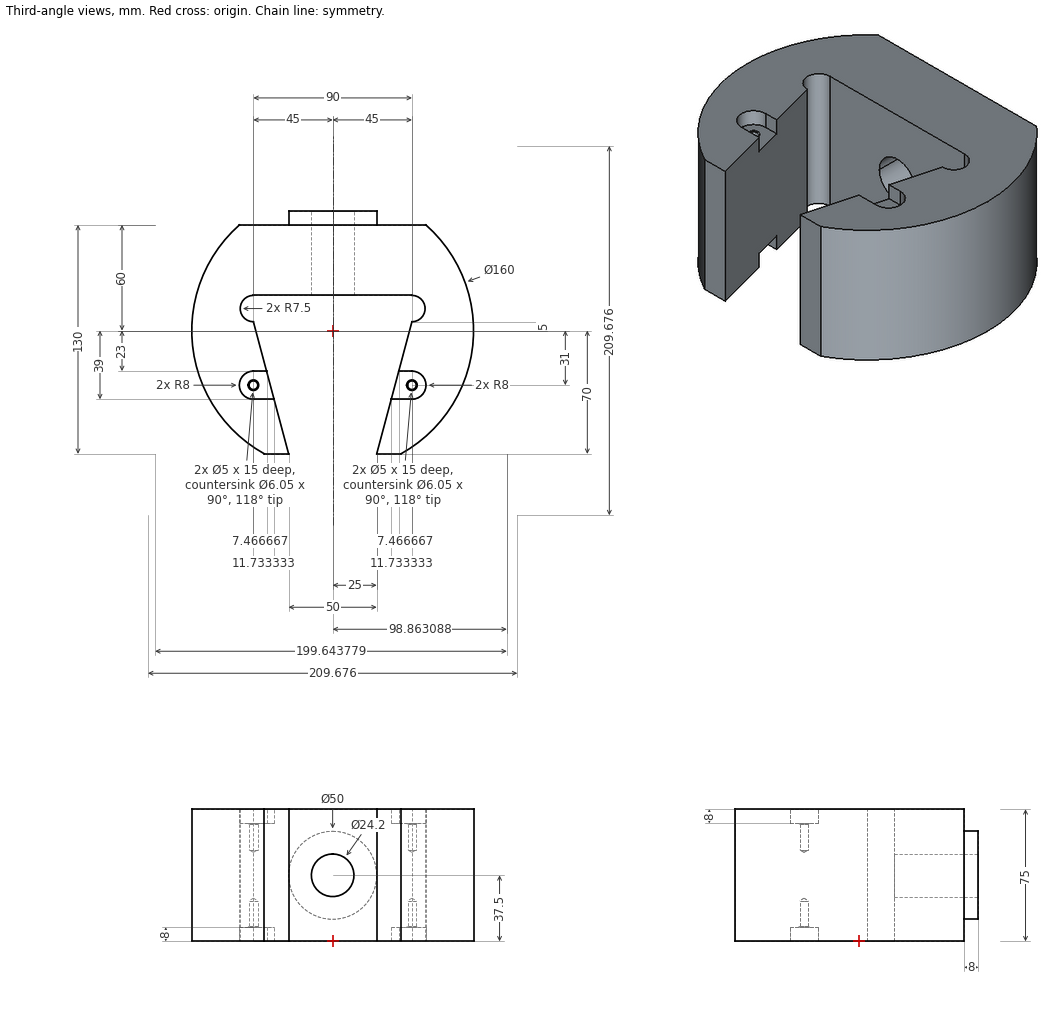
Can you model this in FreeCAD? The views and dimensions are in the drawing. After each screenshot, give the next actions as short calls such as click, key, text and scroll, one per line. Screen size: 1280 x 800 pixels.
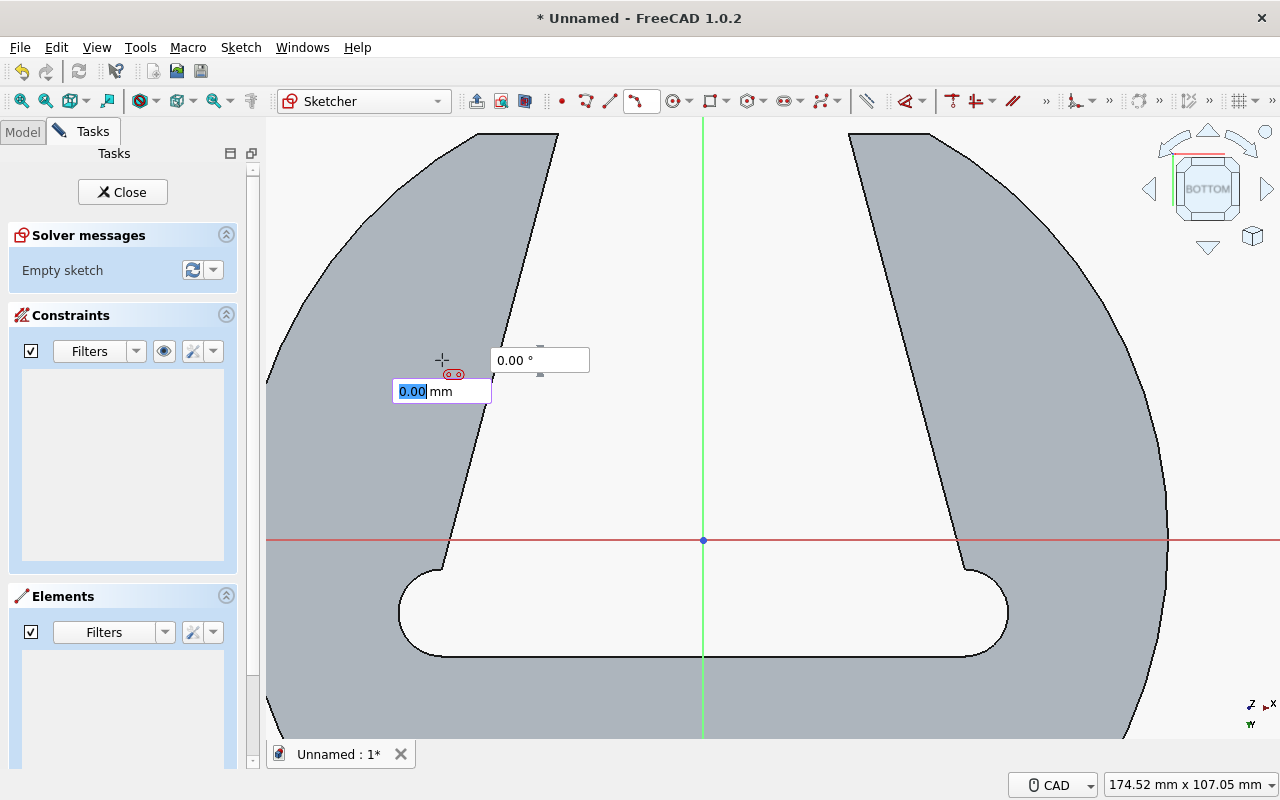
click(965, 360)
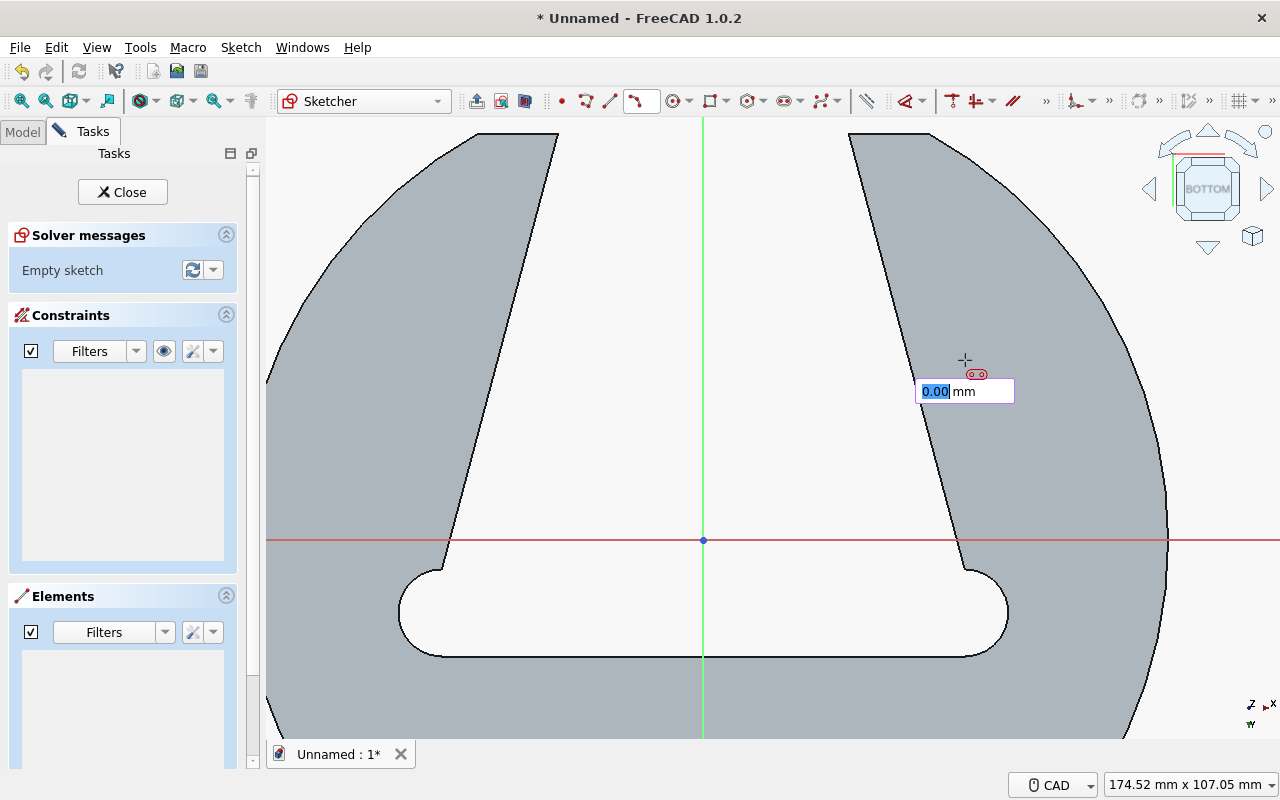
click(625, 407)
key(Escape)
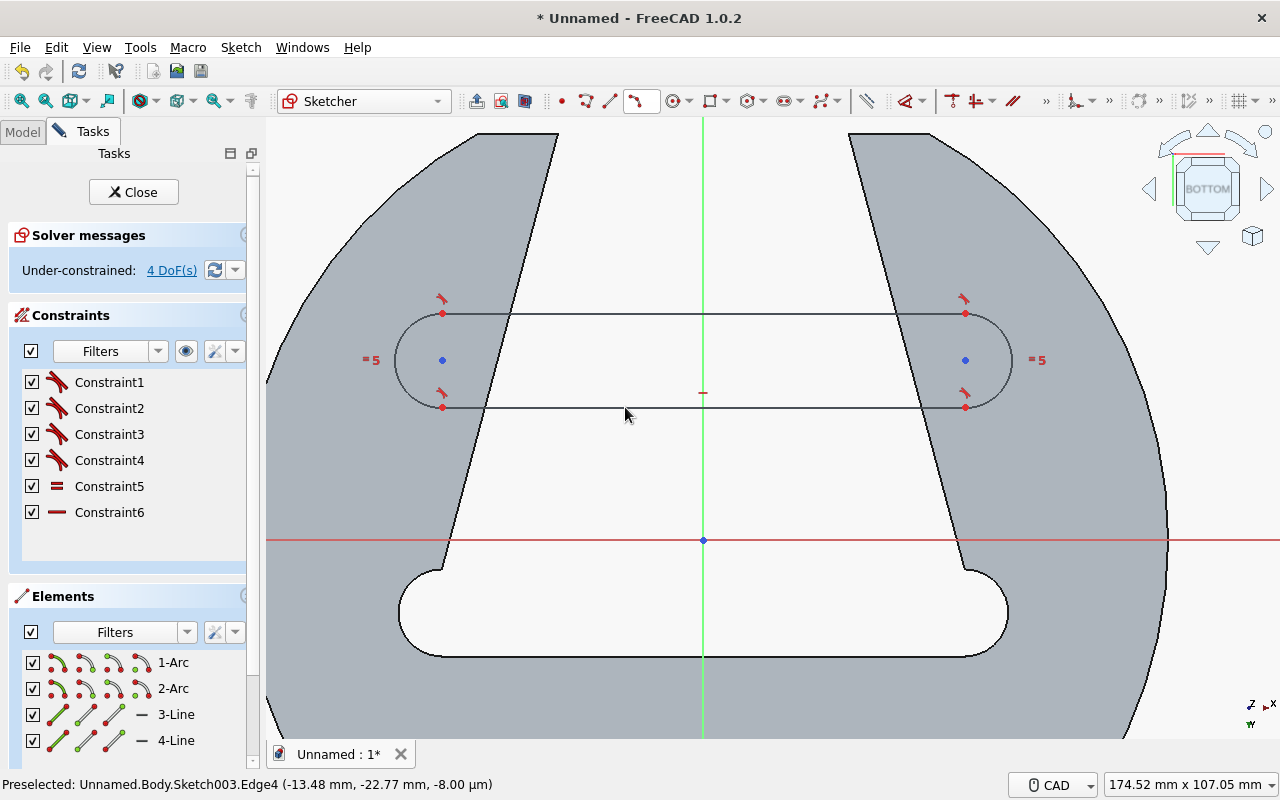
key(d)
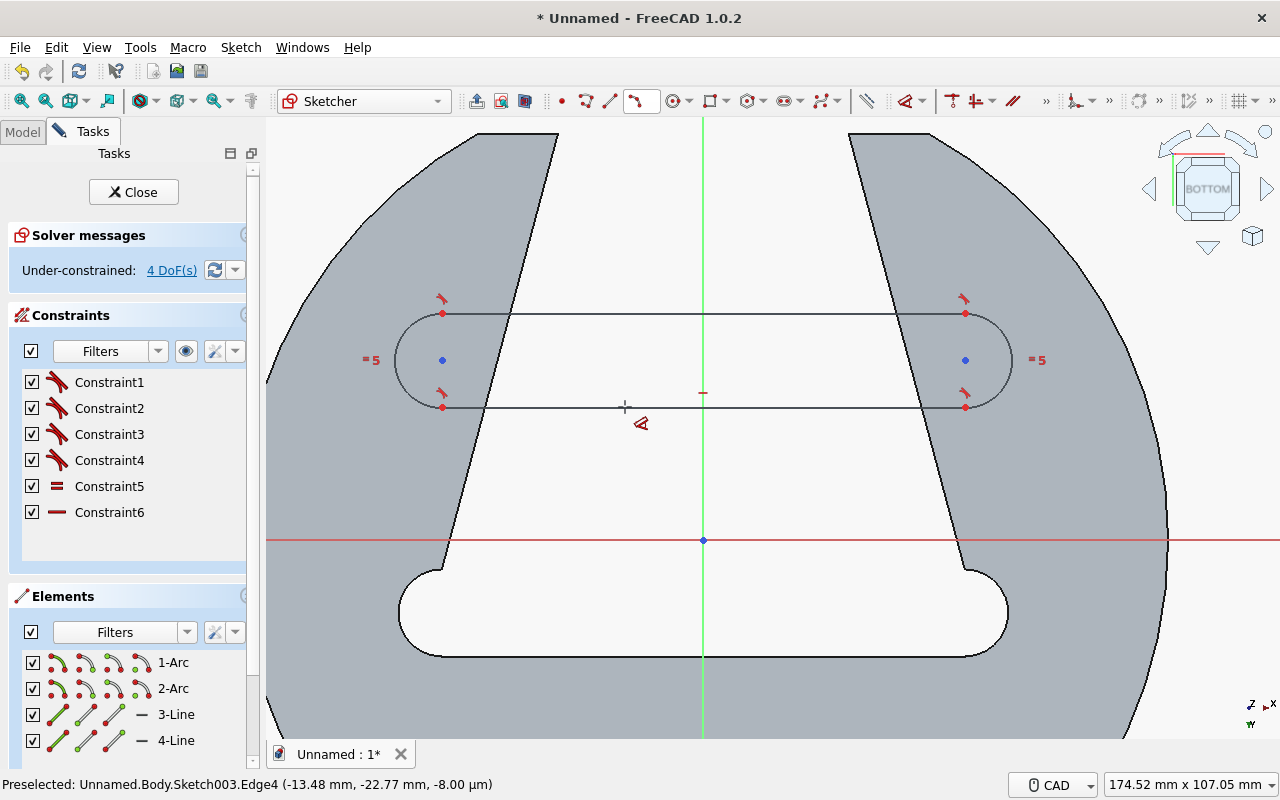
click(404, 333)
click(378, 314)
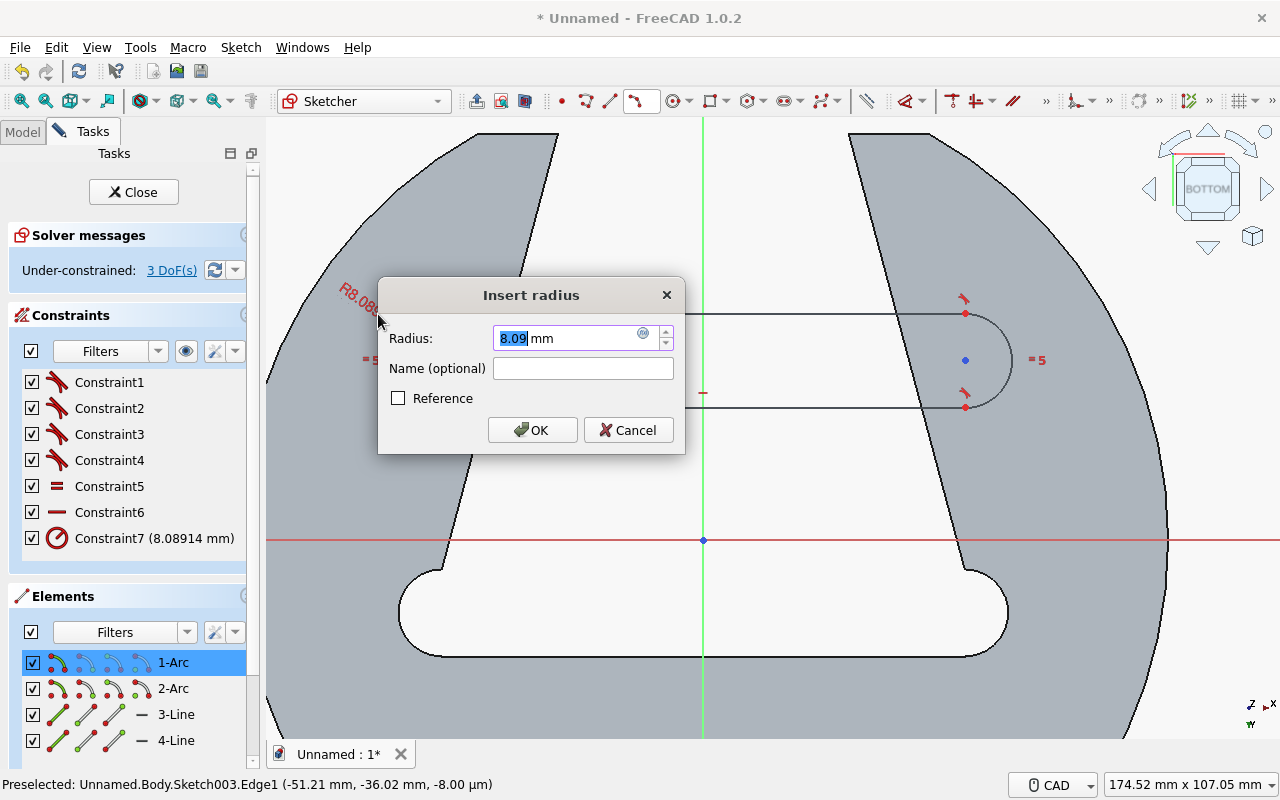
text(8)
key(Return)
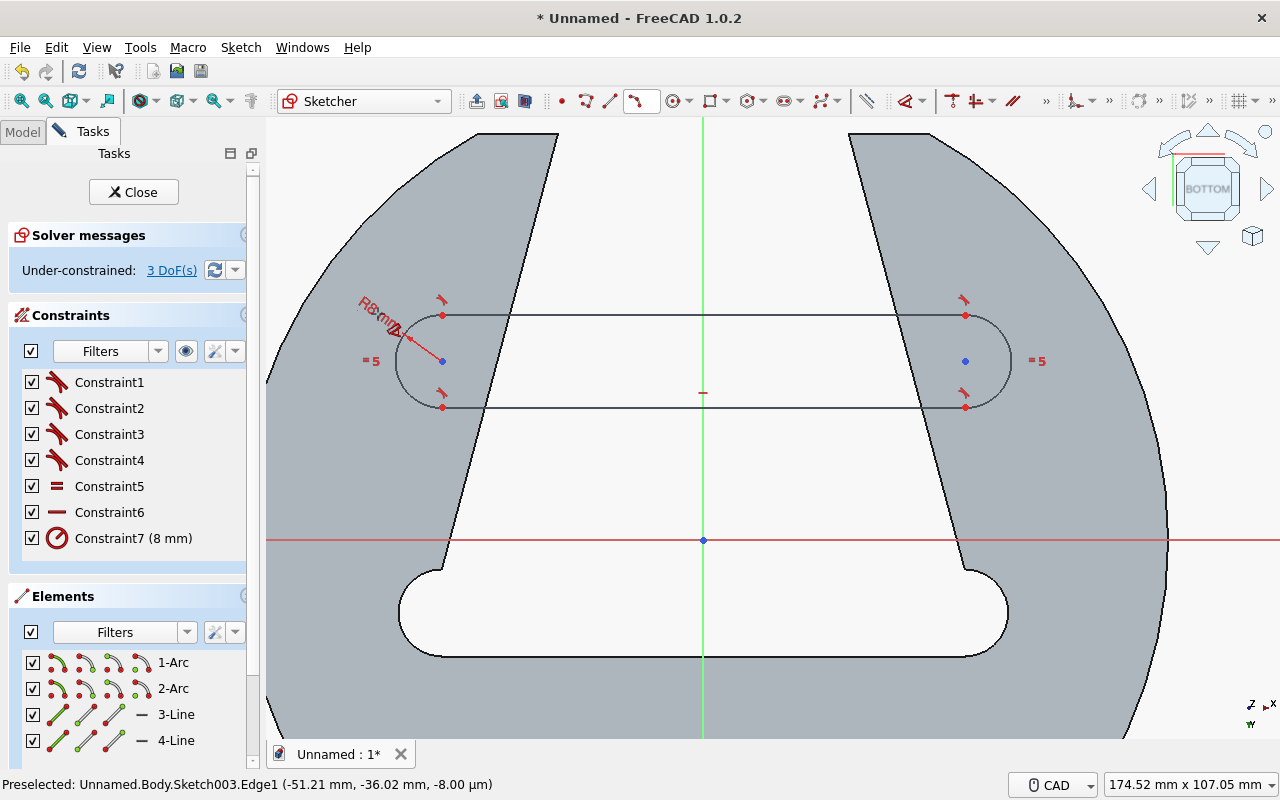
click(599, 315)
click(583, 281)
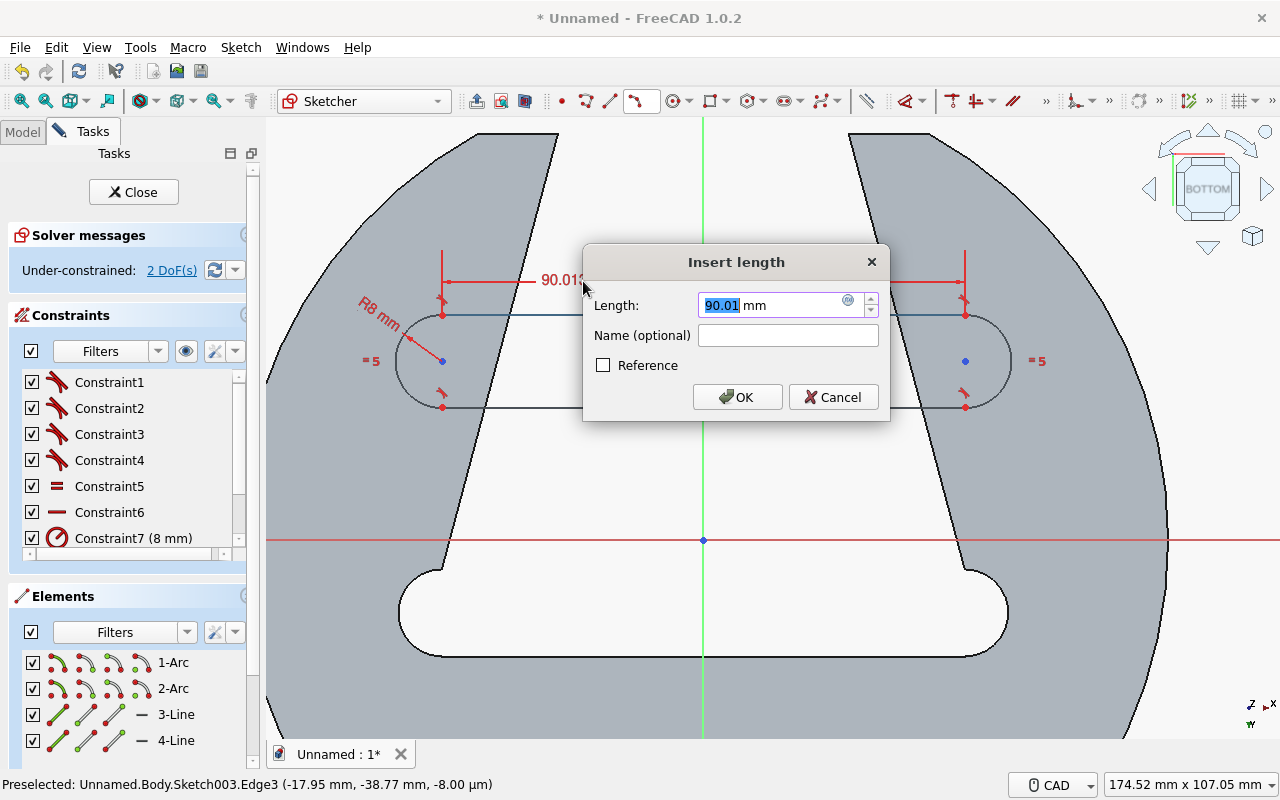
text(90)
key(Return)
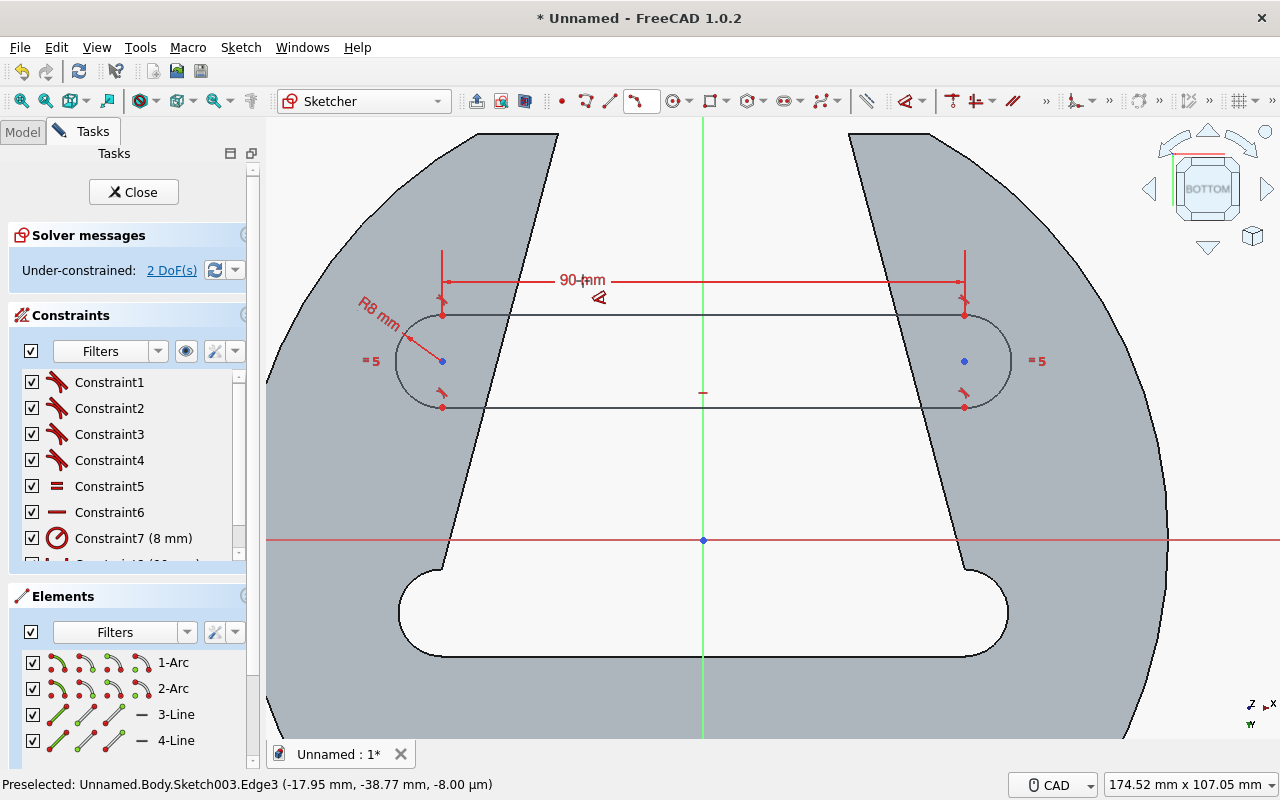
click(442, 315)
click(573, 574)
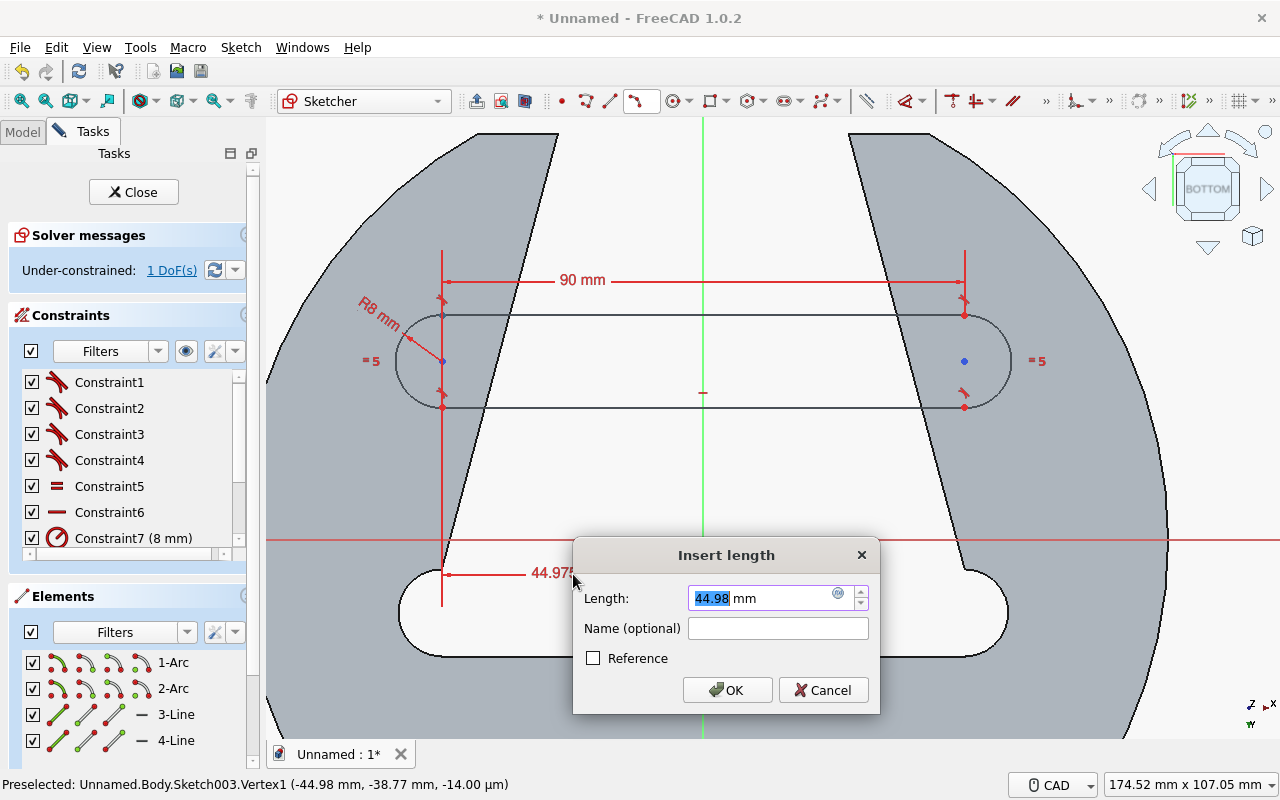
text(45)
key(Return)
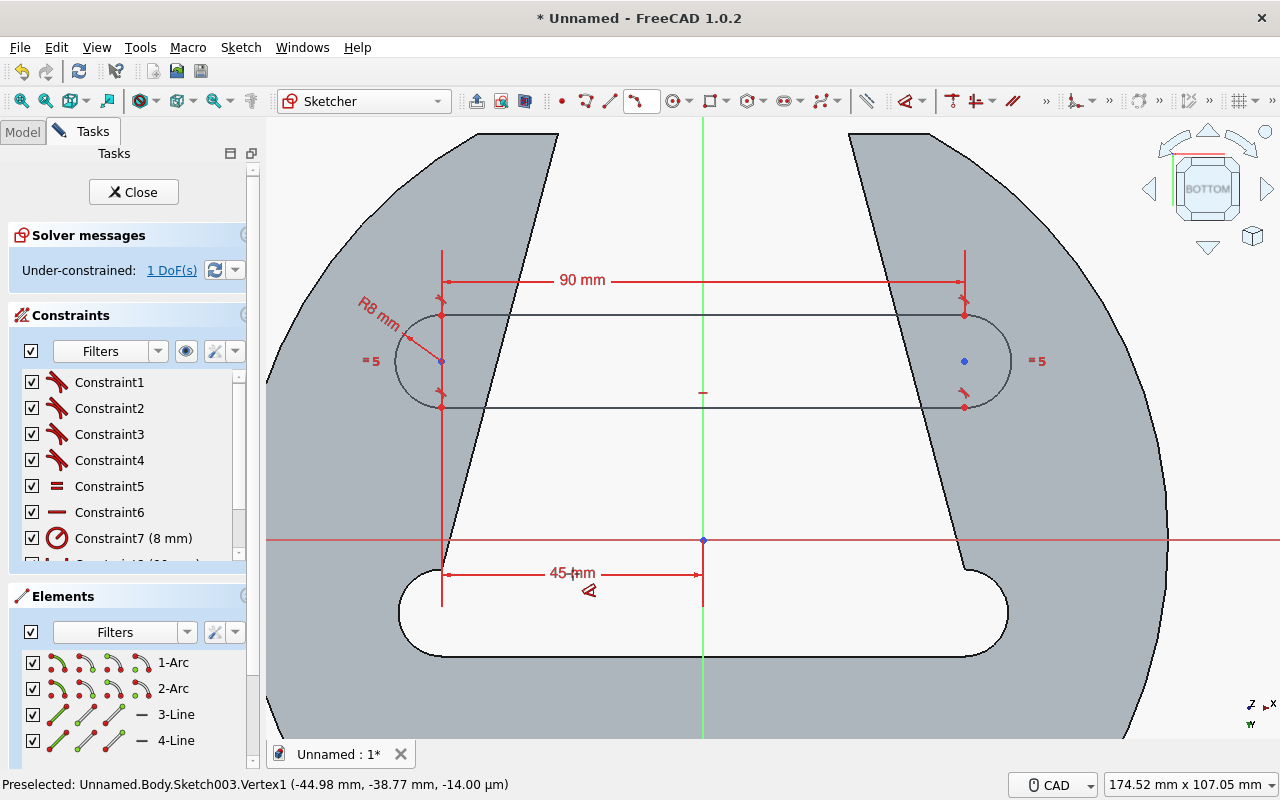
click(442, 315)
click(408, 428)